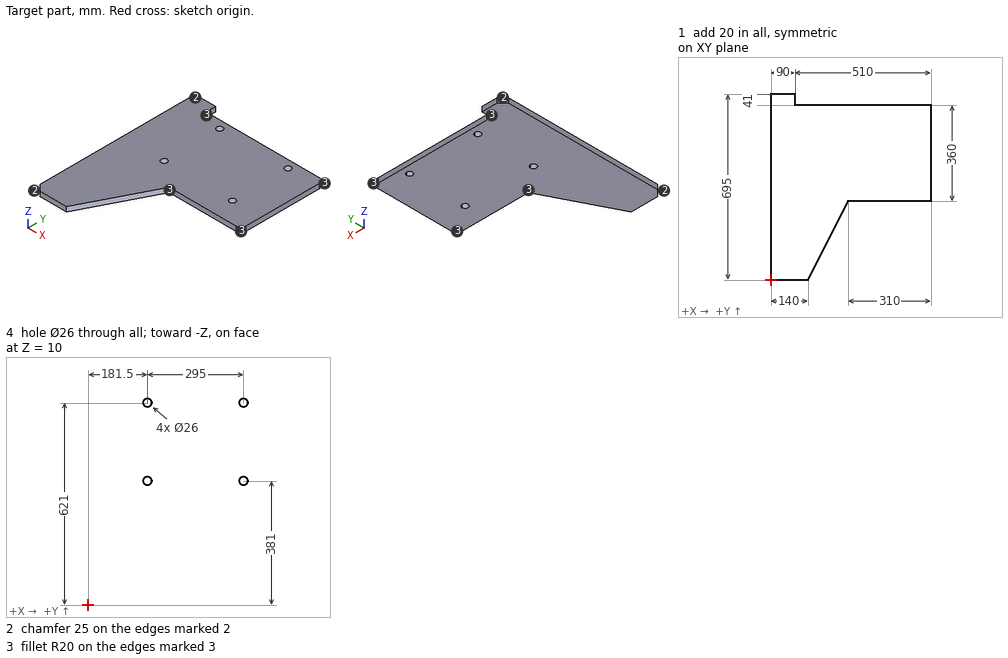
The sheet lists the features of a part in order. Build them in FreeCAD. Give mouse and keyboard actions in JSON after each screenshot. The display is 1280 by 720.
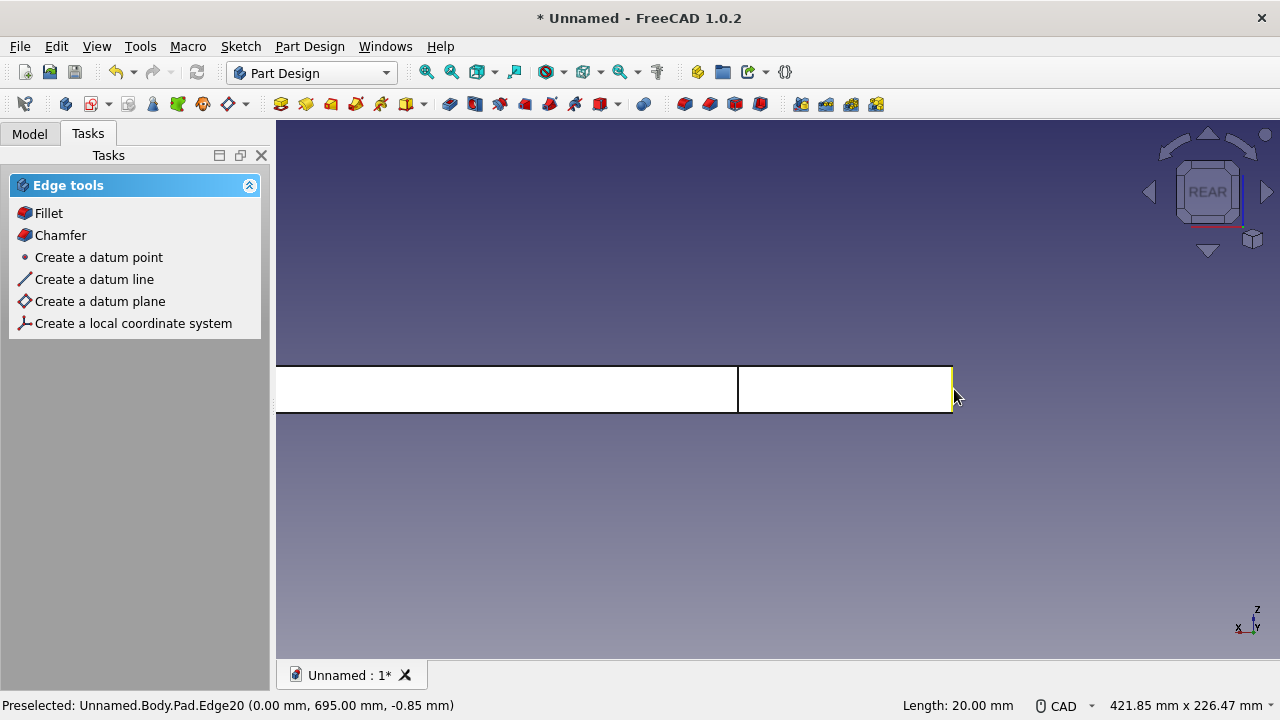
{"action": "left_click", "coordinate": [952, 389], "text": "ctrl"}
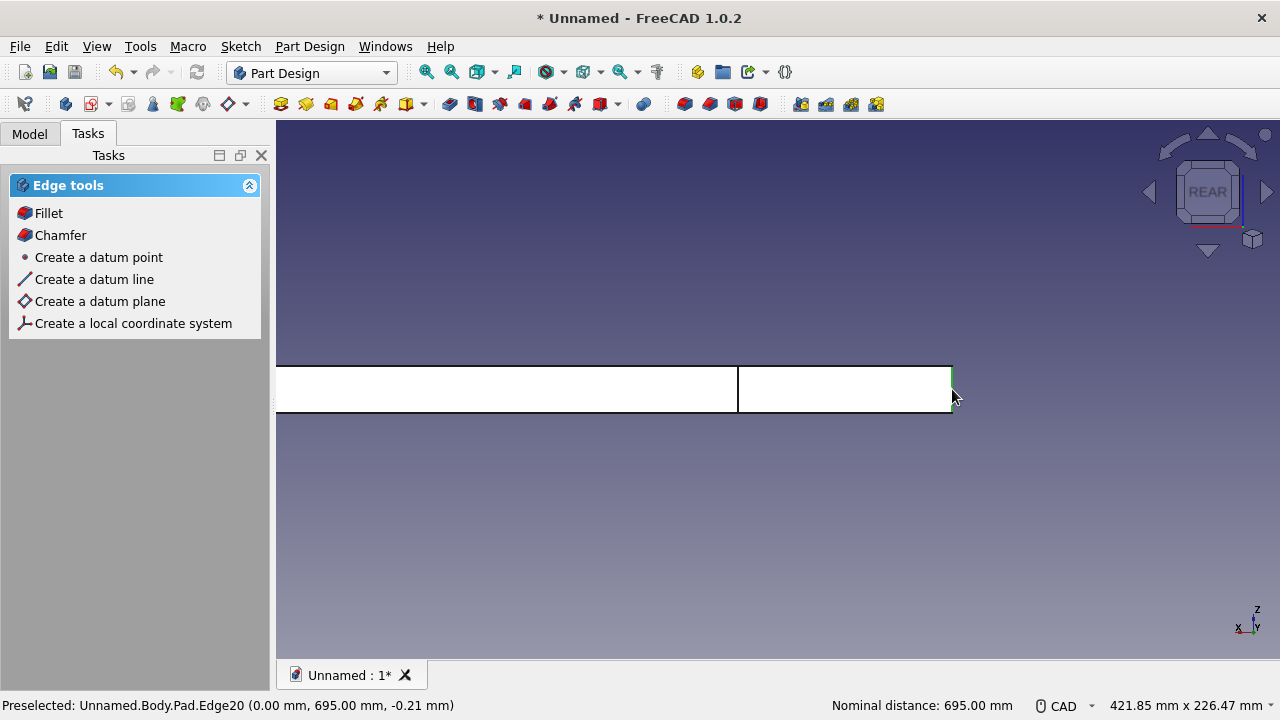
{"action": "left_click", "coordinate": [710, 104]}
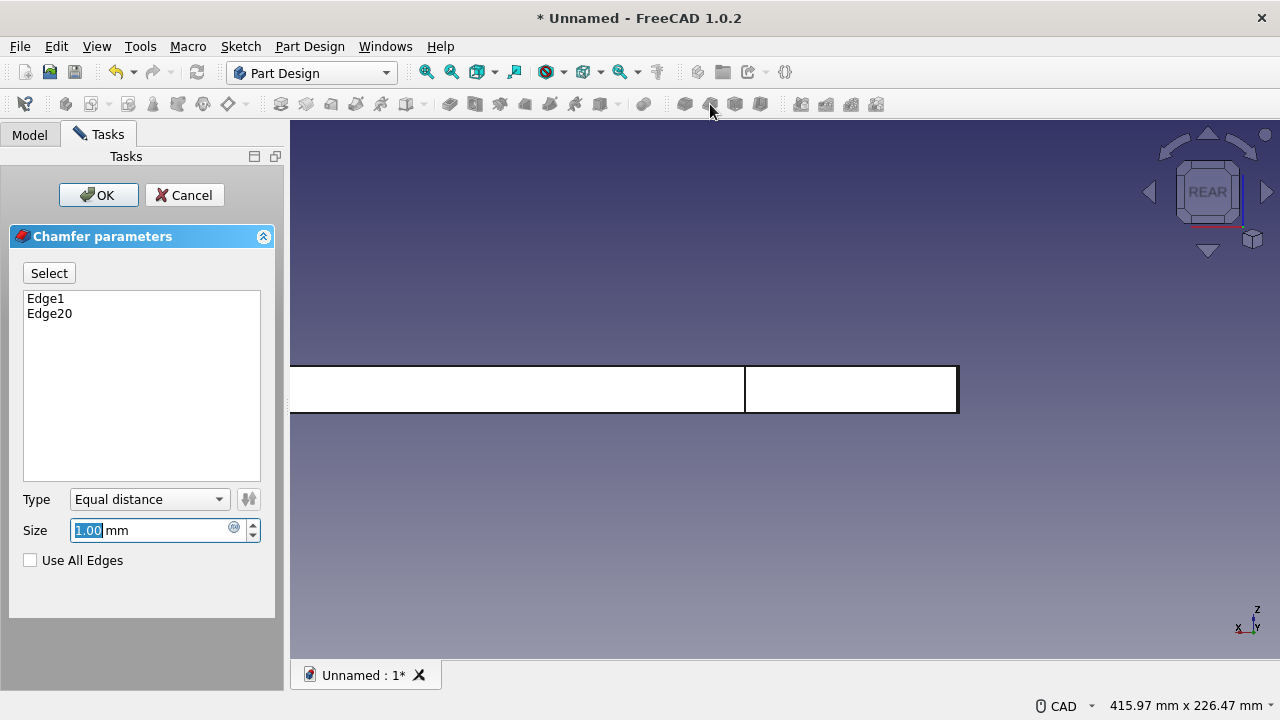
{"action": "type", "text": "25"}
{"action": "key", "text": "Tab"}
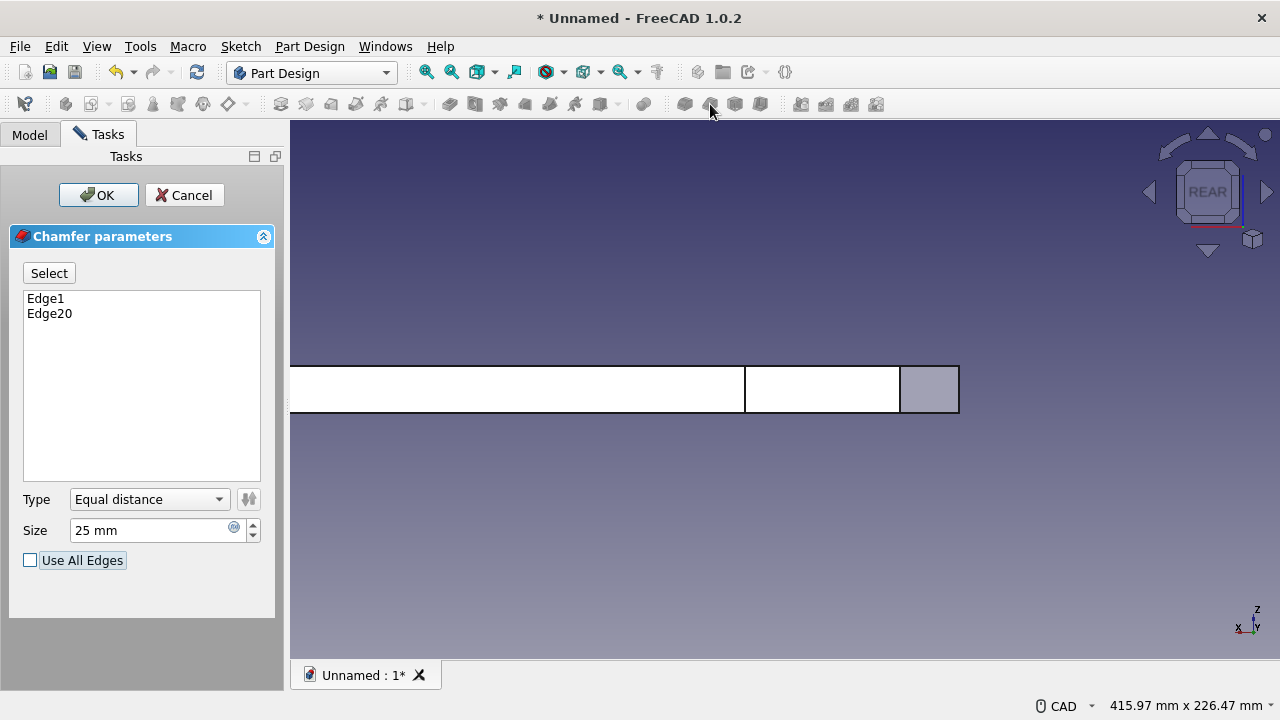
{"action": "left_click", "coordinate": [99, 195]}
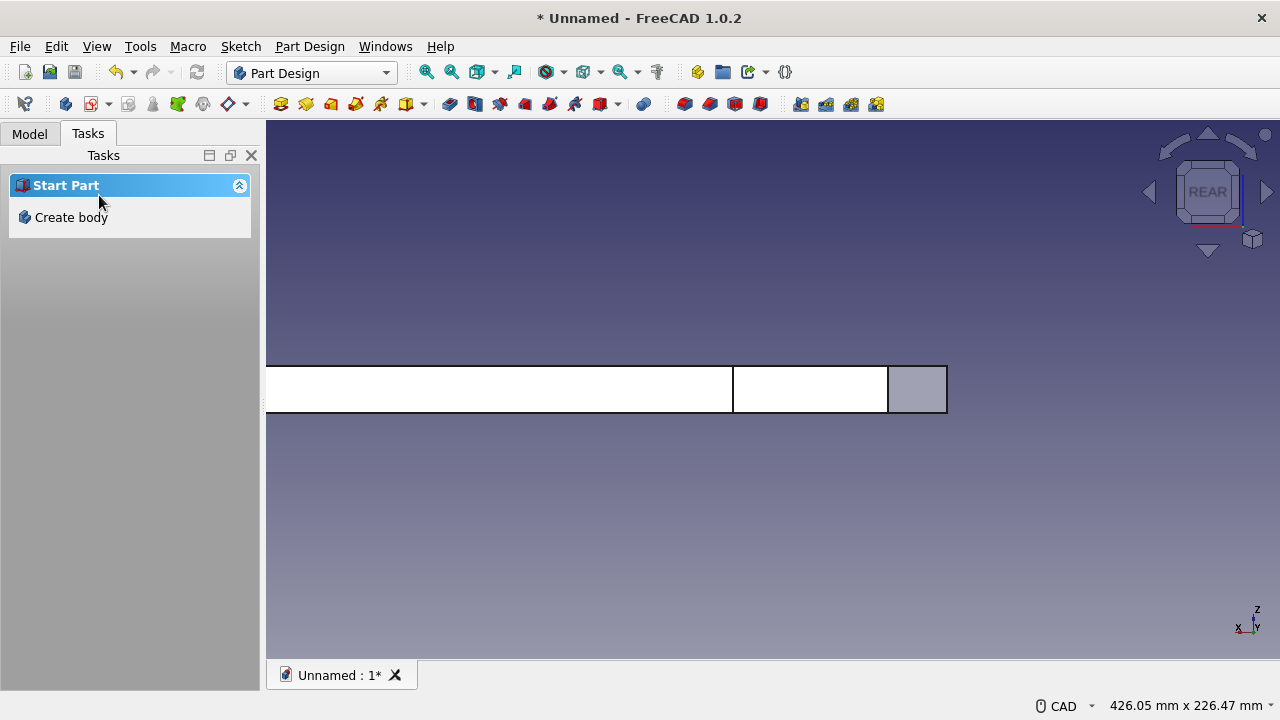
{"action": "left_click", "coordinate": [427, 72]}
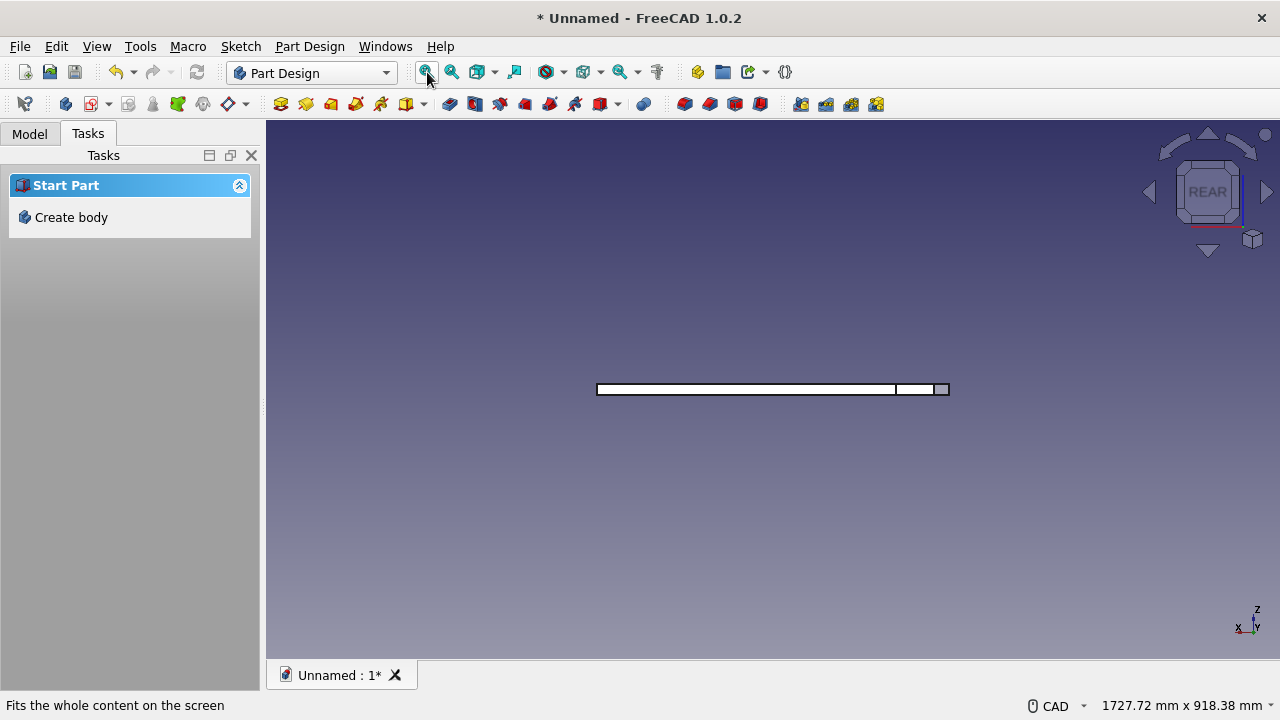
{"action": "scroll", "coordinate": [896, 389], "scroll_direction": "up", "scroll_amount": 7}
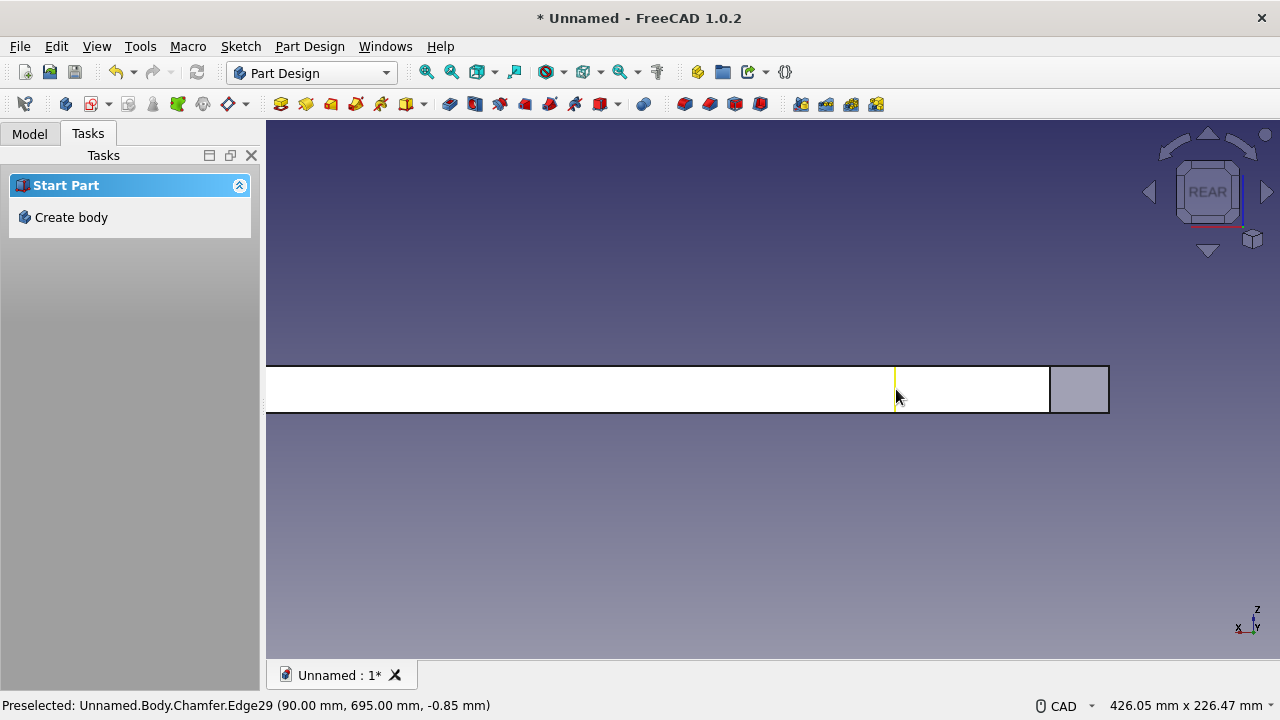
{"action": "left_click", "coordinate": [427, 72]}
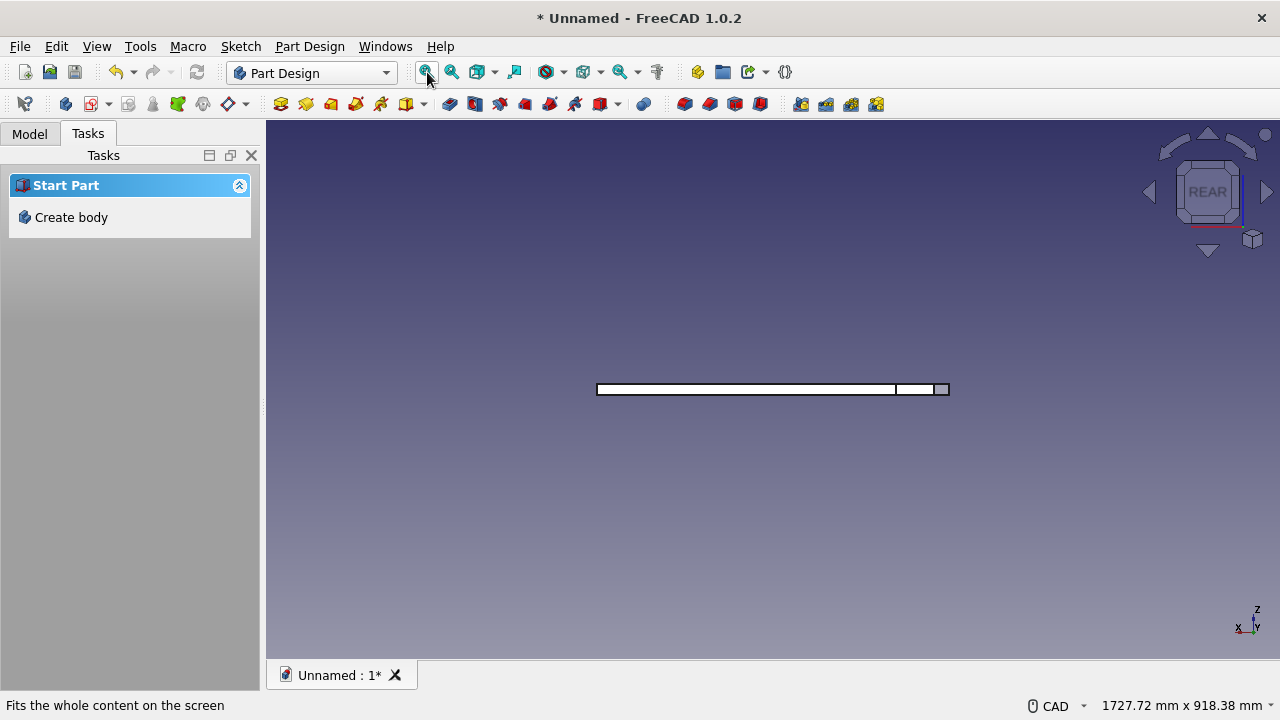
{"action": "key", "text": "0"}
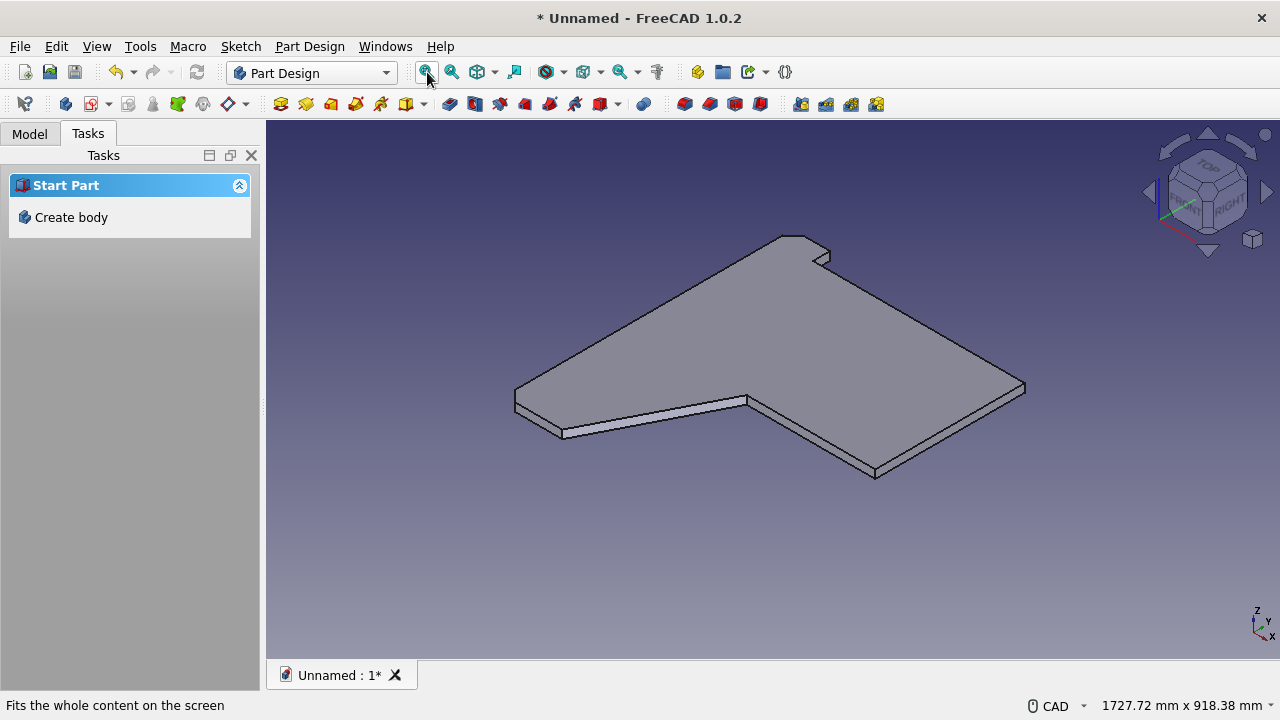
{"action": "left_click", "coordinate": [875, 475]}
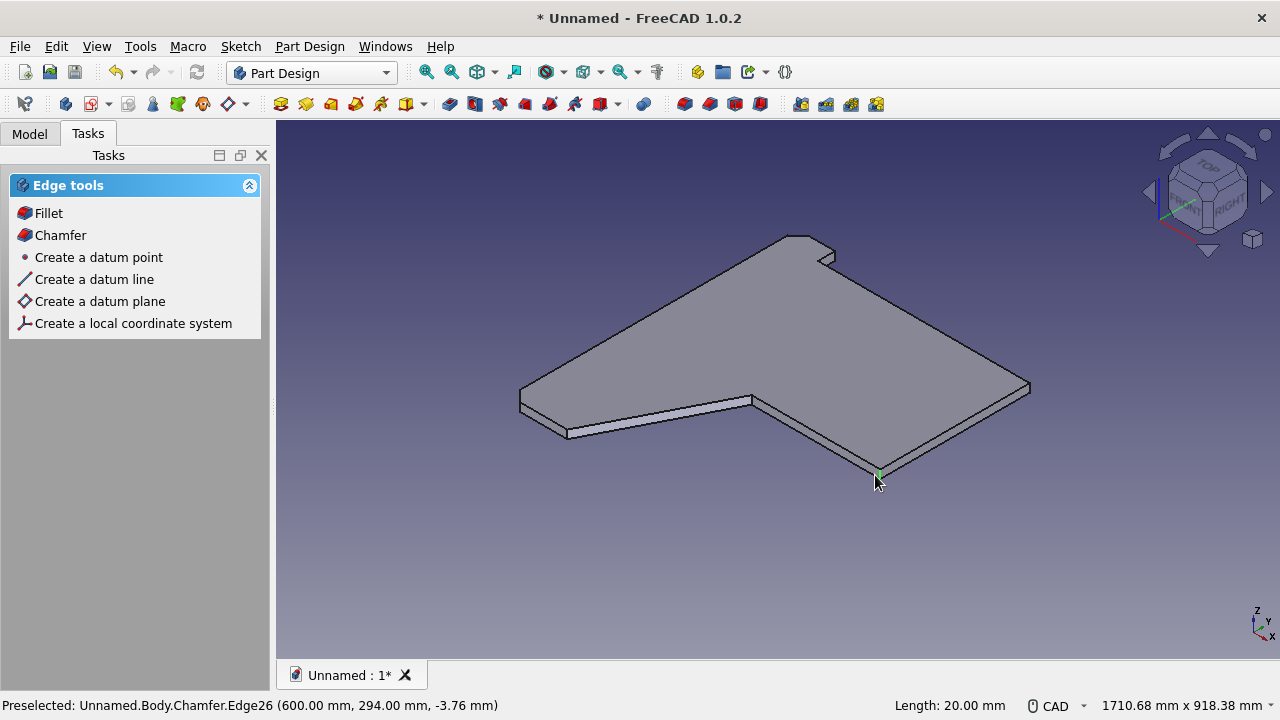
{"action": "scroll", "coordinate": [818, 265], "scroll_direction": "up", "scroll_amount": 7}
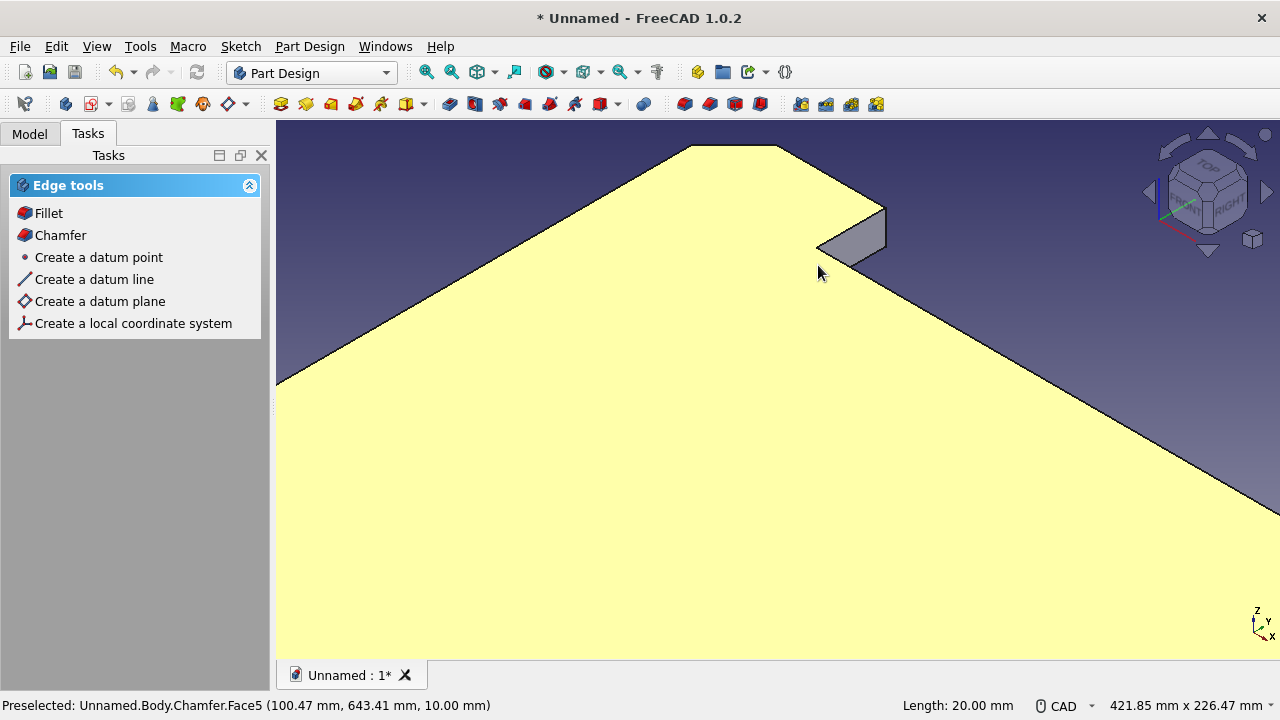
{"action": "left_click", "coordinate": [427, 72]}